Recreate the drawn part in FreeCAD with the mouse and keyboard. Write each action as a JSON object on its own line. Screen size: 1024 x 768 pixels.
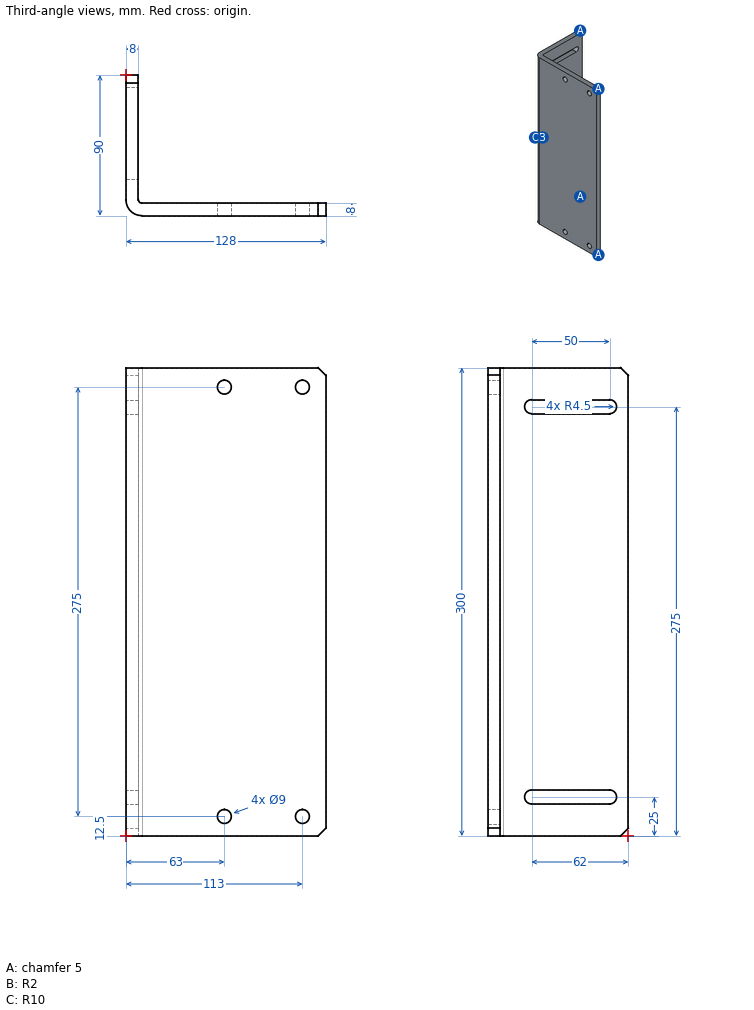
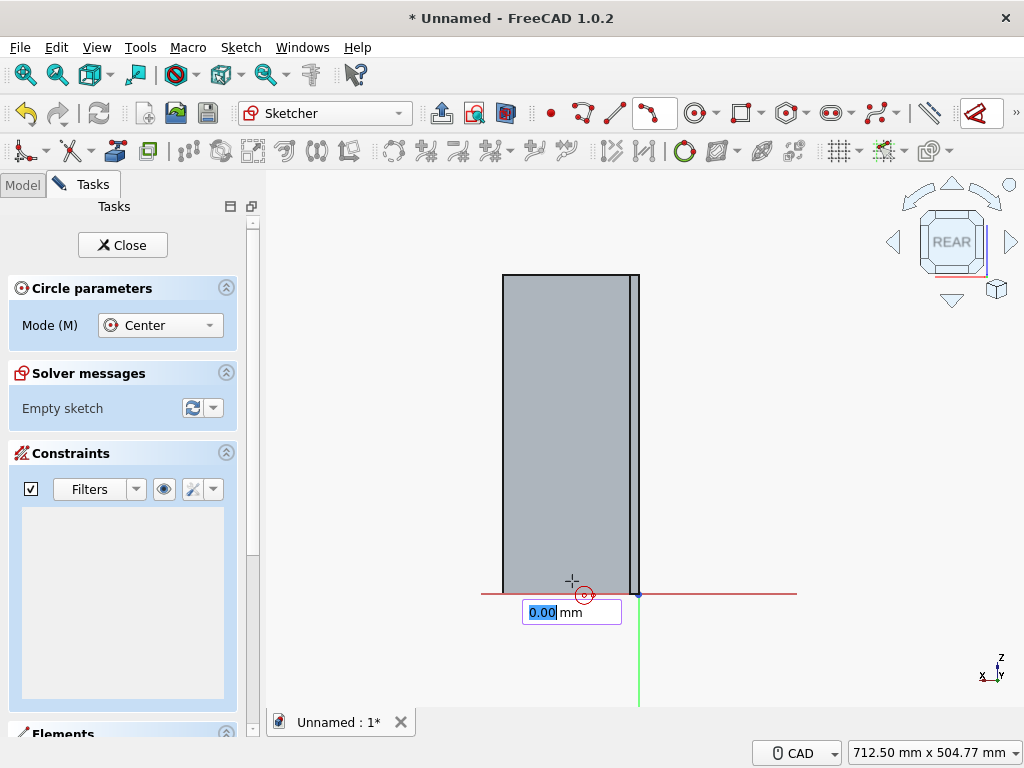
{"action": "scroll", "coordinate": [575, 577], "scroll_direction": "up", "scroll_amount": 6}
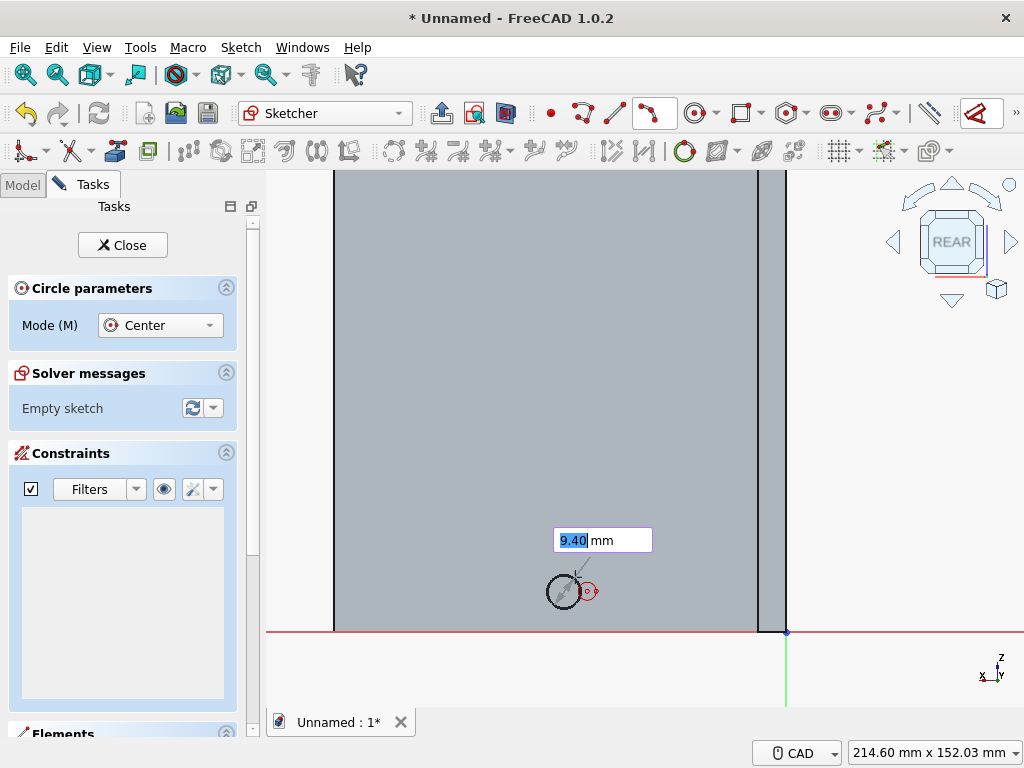
{"action": "left_click", "coordinate": [575, 577]}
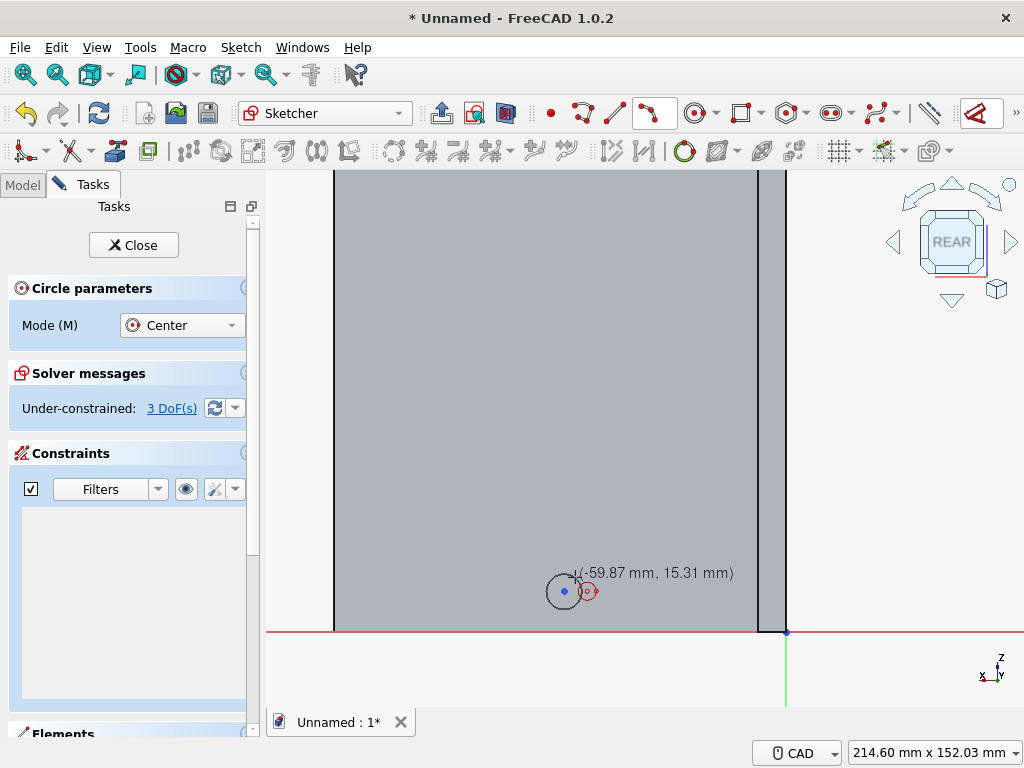
{"action": "scroll", "coordinate": [387, 588], "scroll_direction": "up", "scroll_amount": 2}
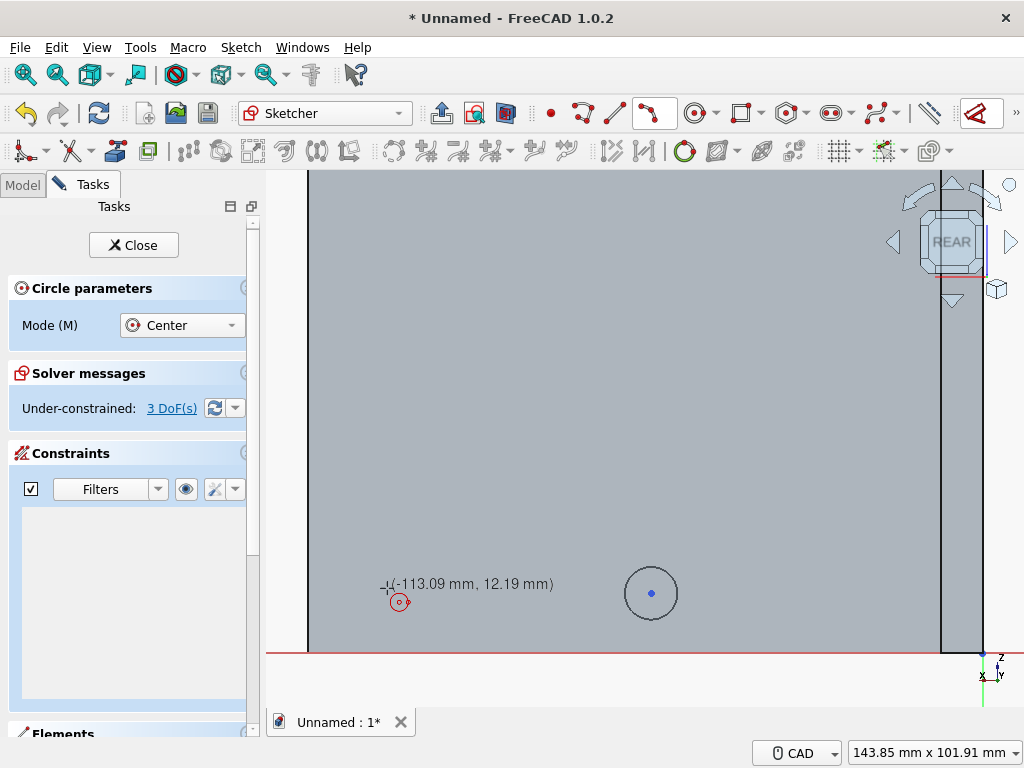
{"action": "scroll", "coordinate": [552, 579], "scroll_direction": "down", "scroll_amount": 8}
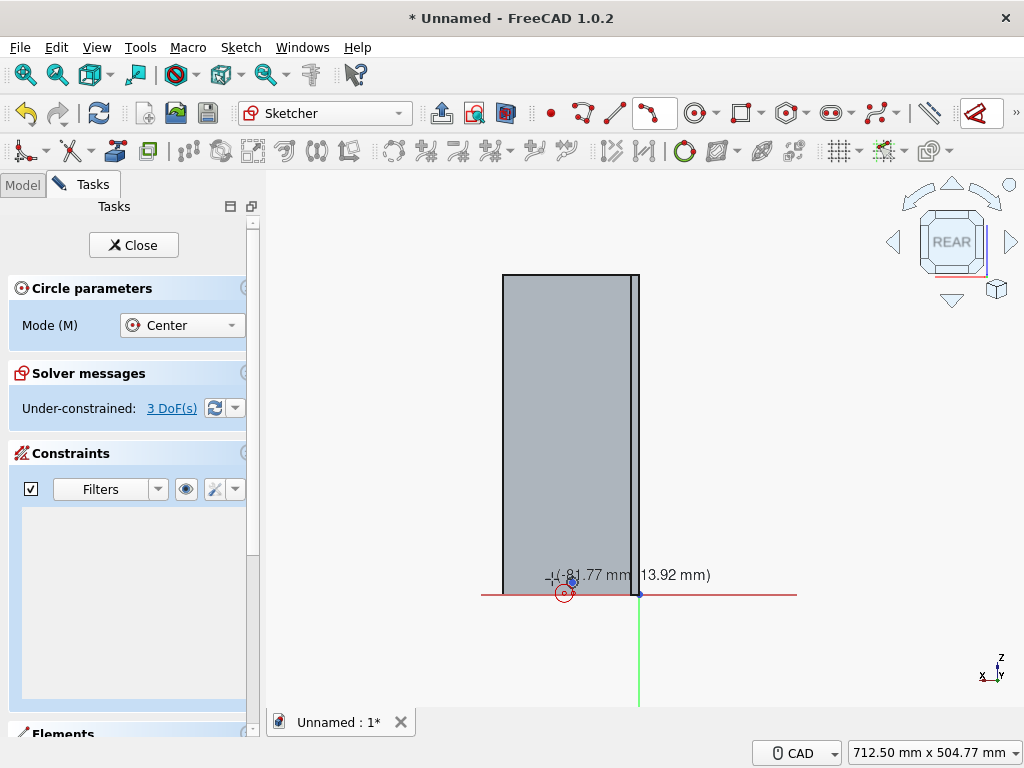
{"action": "left_click", "coordinate": [519, 581]}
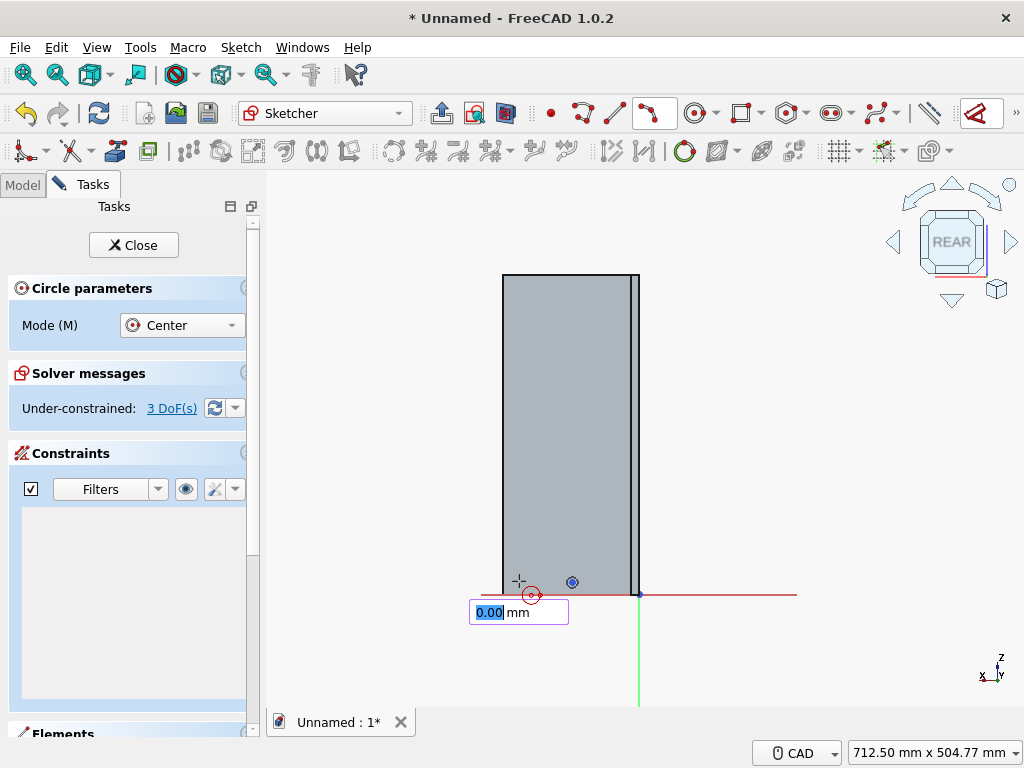
{"action": "scroll", "coordinate": [522, 578], "scroll_direction": "up", "scroll_amount": 6}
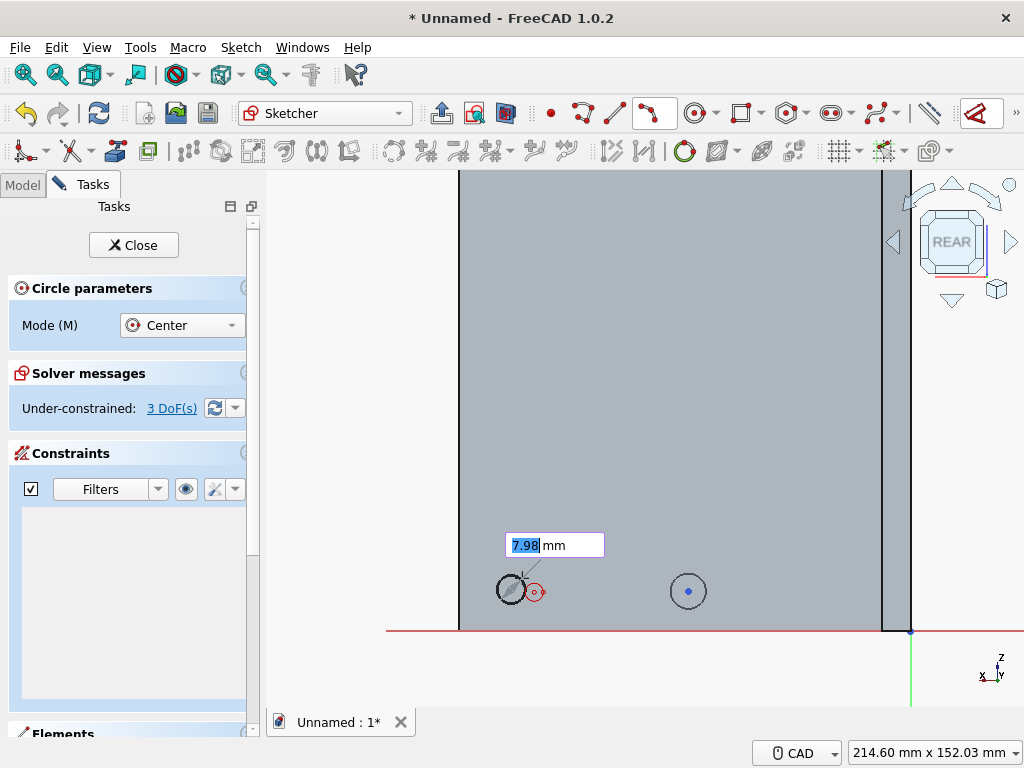
{"action": "left_click", "coordinate": [523, 576]}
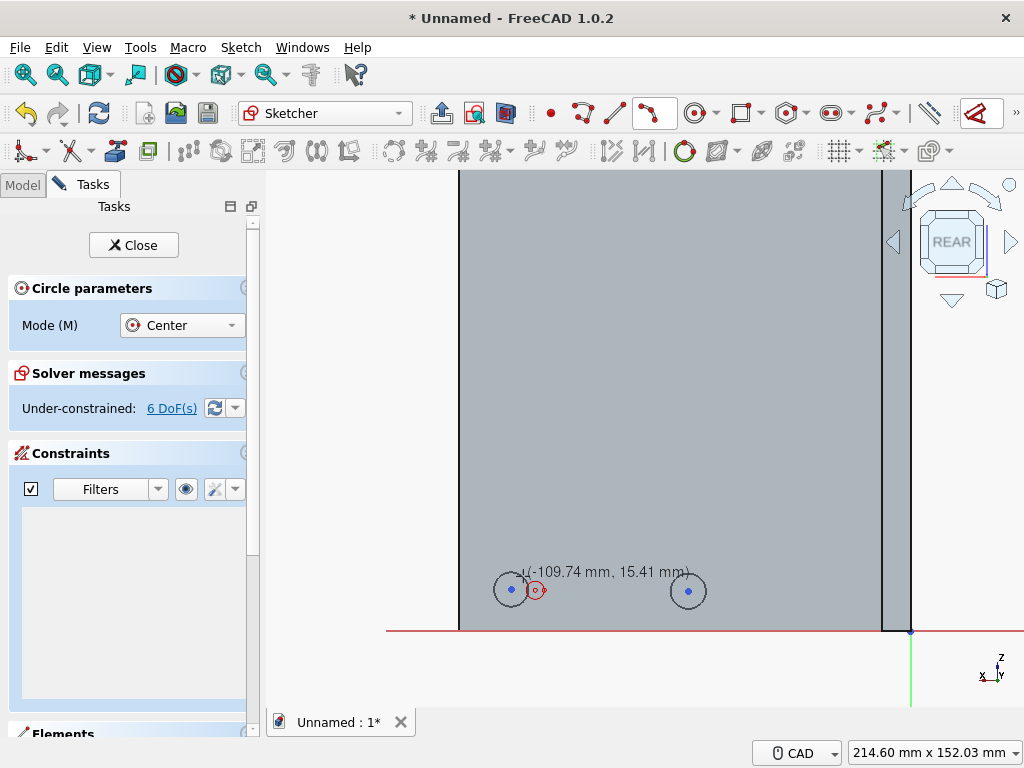
{"action": "scroll", "coordinate": [522, 578], "scroll_direction": "down", "scroll_amount": 6}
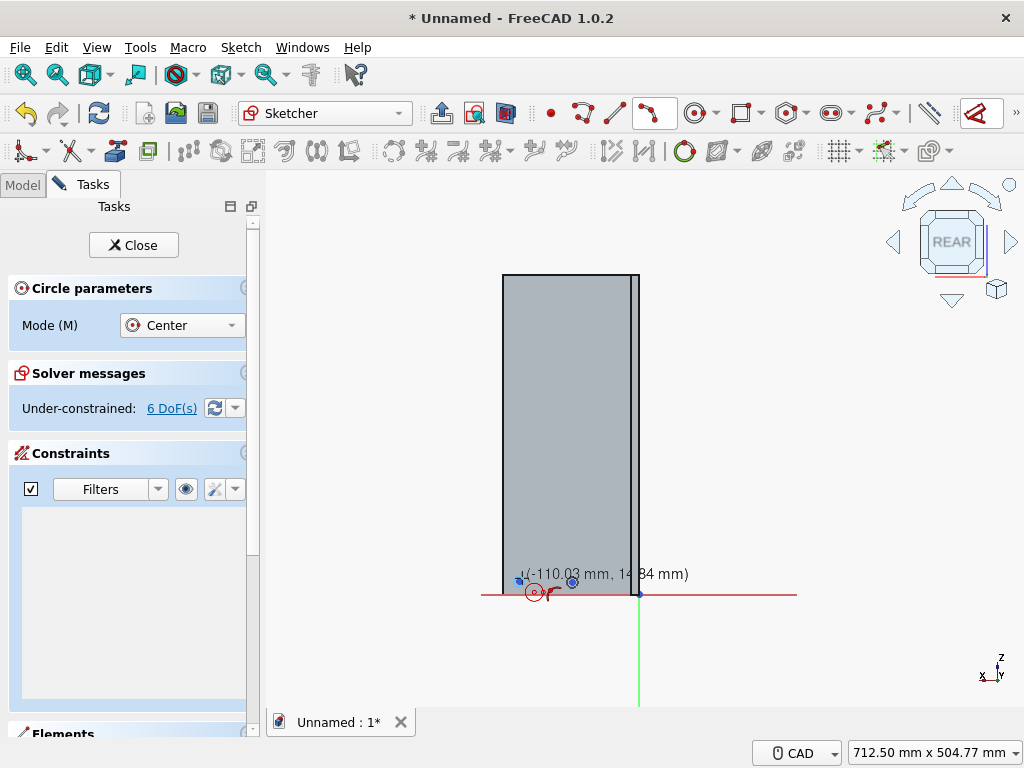
{"action": "scroll", "coordinate": [572, 289], "scroll_direction": "up", "scroll_amount": 8}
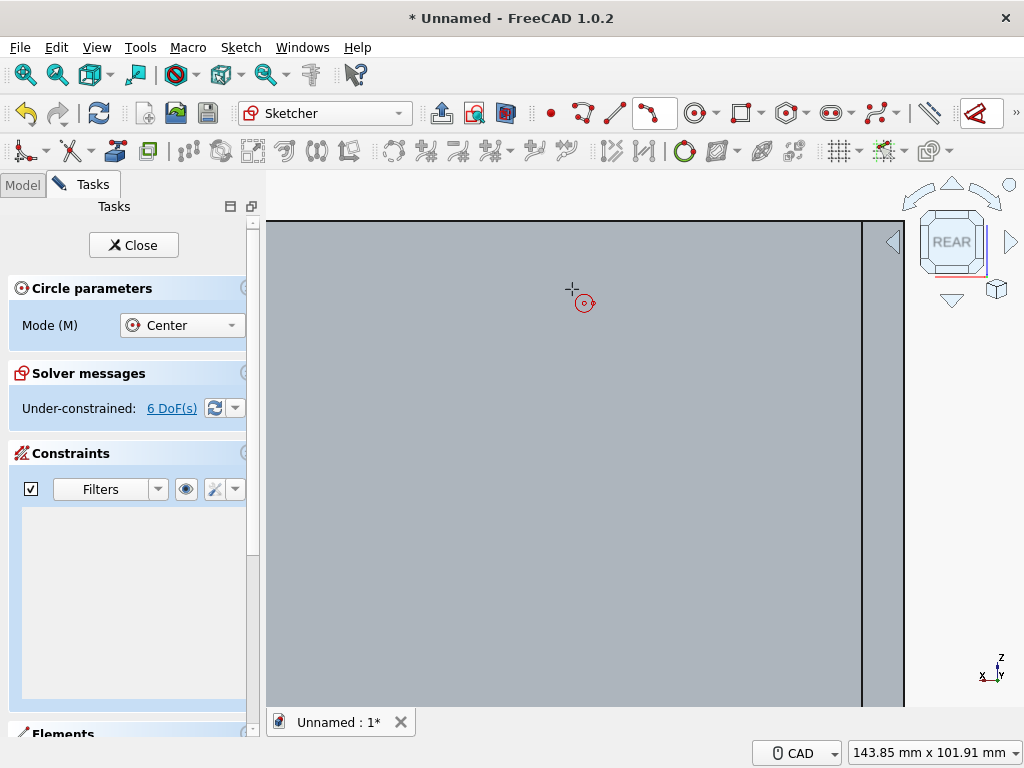
{"action": "scroll", "coordinate": [572, 288], "scroll_direction": "down", "scroll_amount": 8}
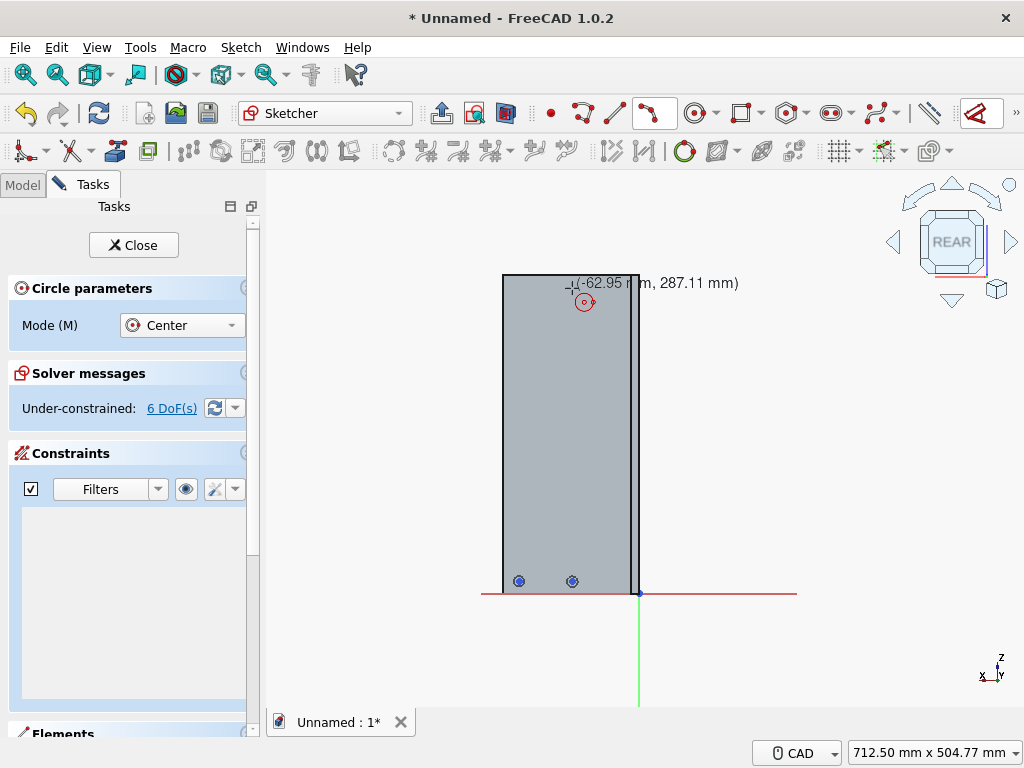
{"action": "left_click", "coordinate": [572, 288]}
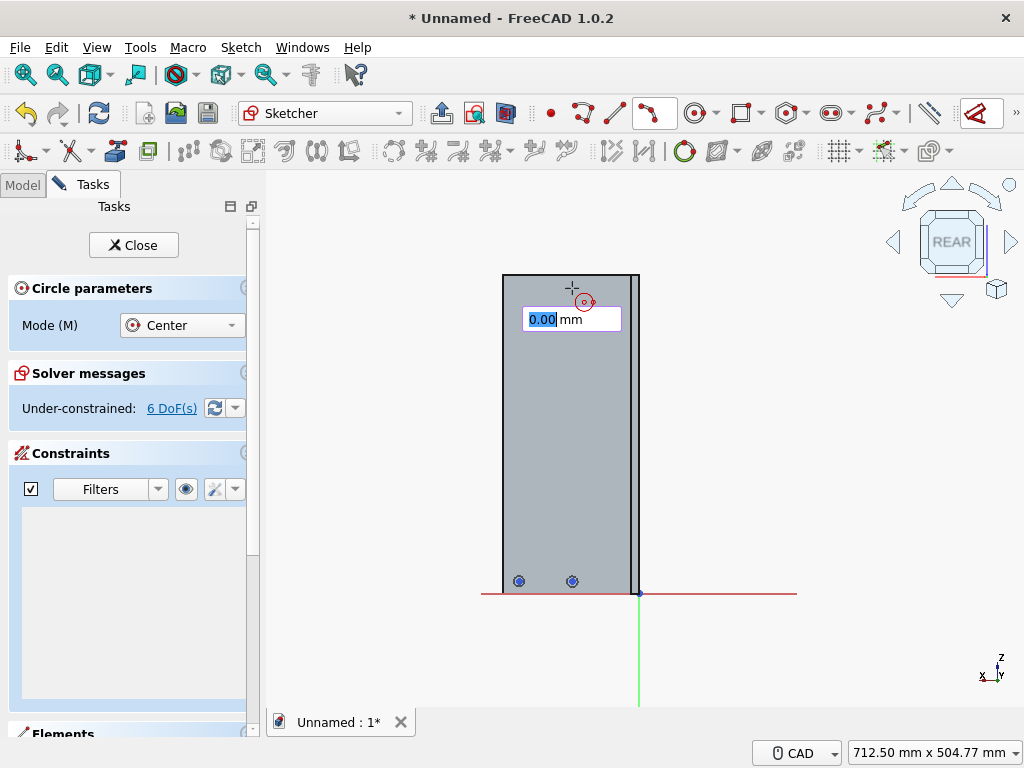
{"action": "scroll", "coordinate": [576, 285], "scroll_direction": "up", "scroll_amount": 6}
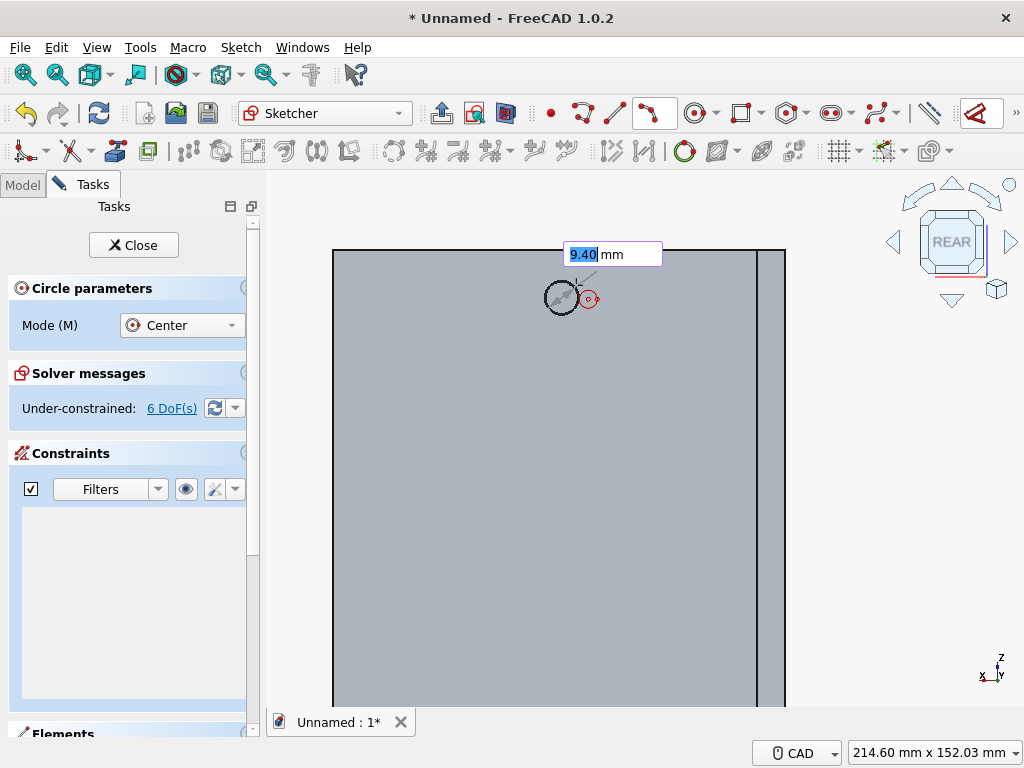
{"action": "left_click", "coordinate": [574, 283]}